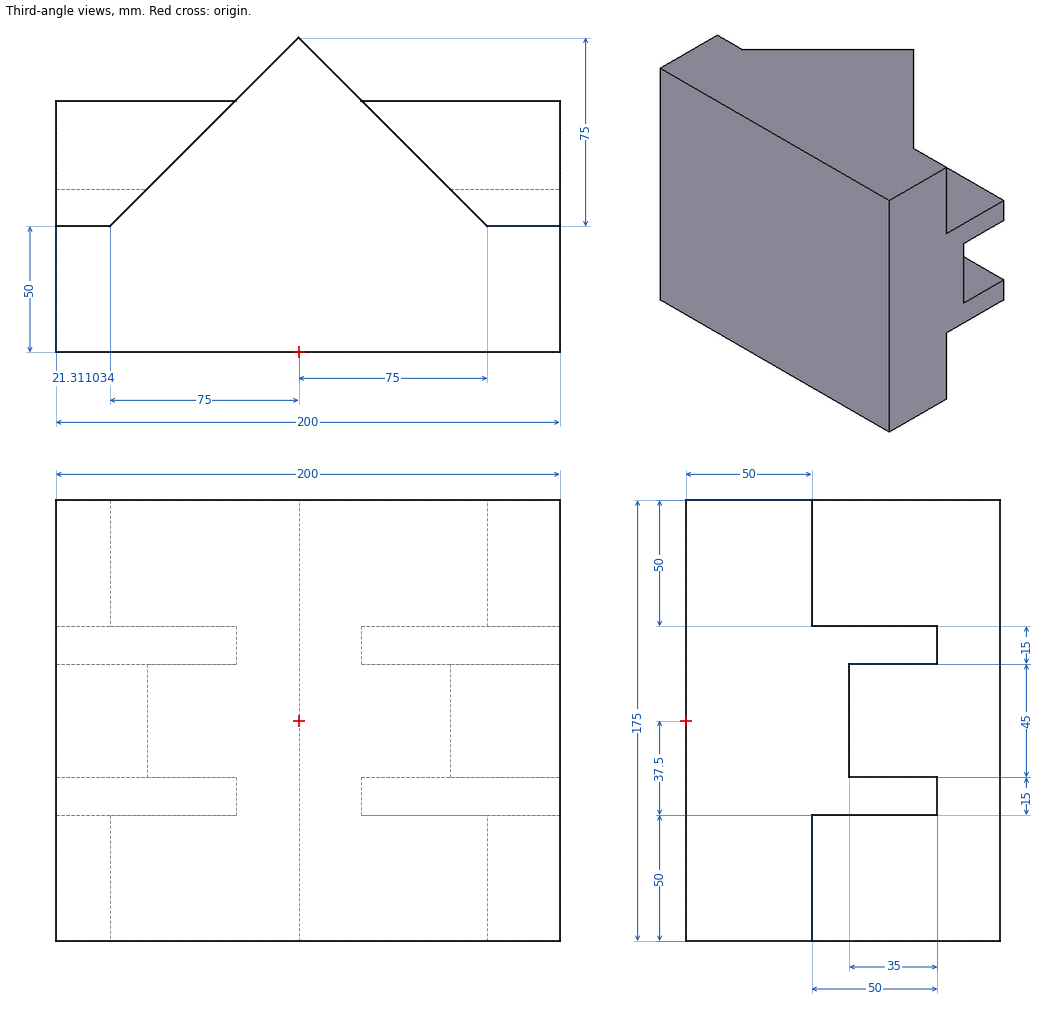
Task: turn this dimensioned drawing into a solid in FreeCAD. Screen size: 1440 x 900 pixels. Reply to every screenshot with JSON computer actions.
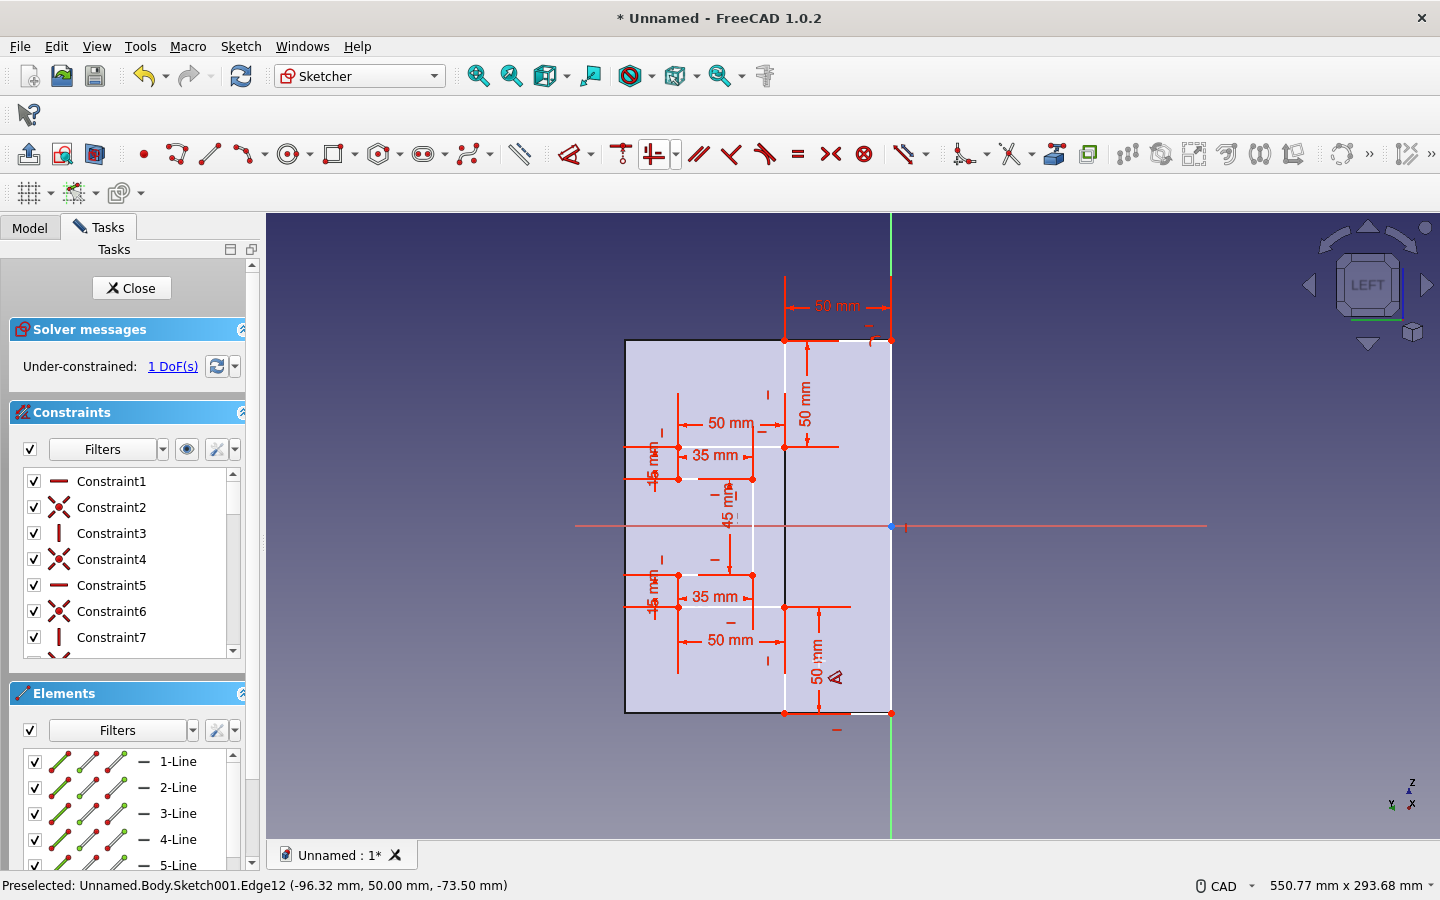
{"action": "left_click", "coordinate": [785, 607]}
{"action": "left_click", "coordinate": [925, 567]}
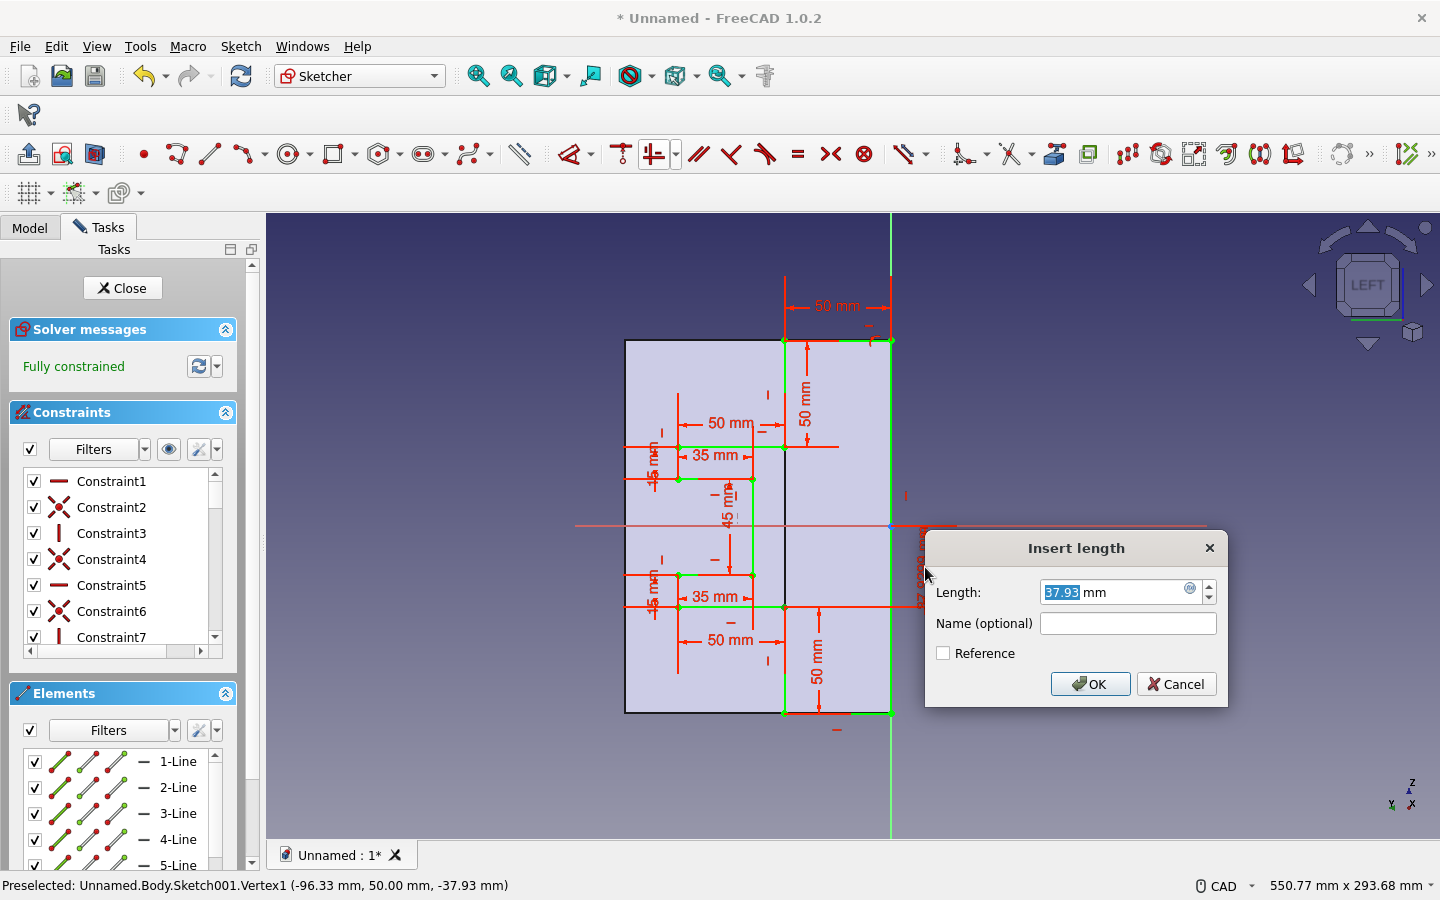
{"action": "type", "text": "37.5"}
{"action": "key", "text": "Return"}
{"action": "key", "text": "Escape"}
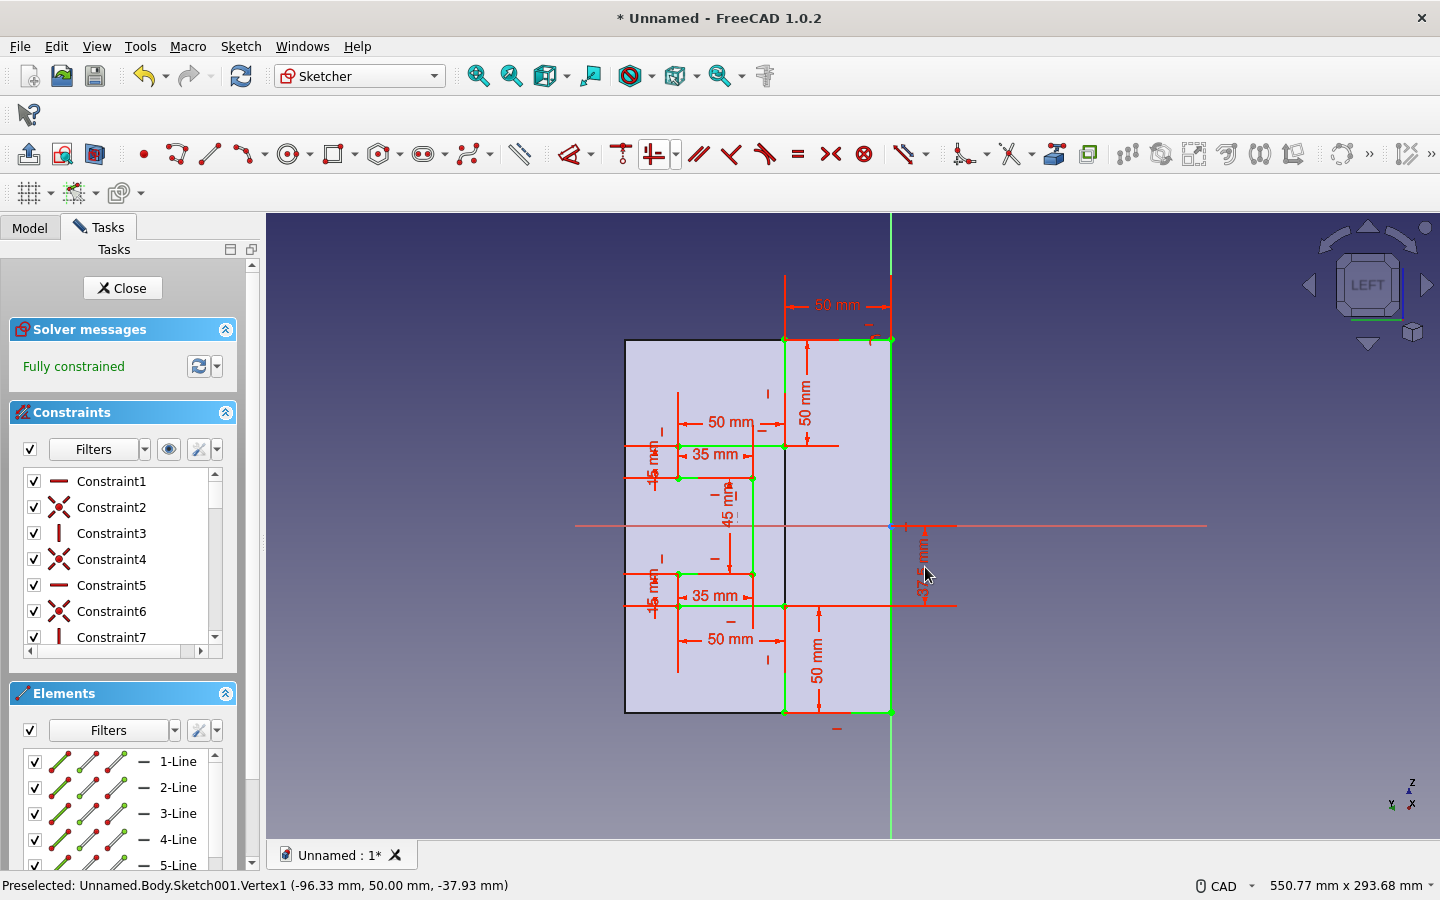
{"action": "left_click", "coordinate": [123, 288]}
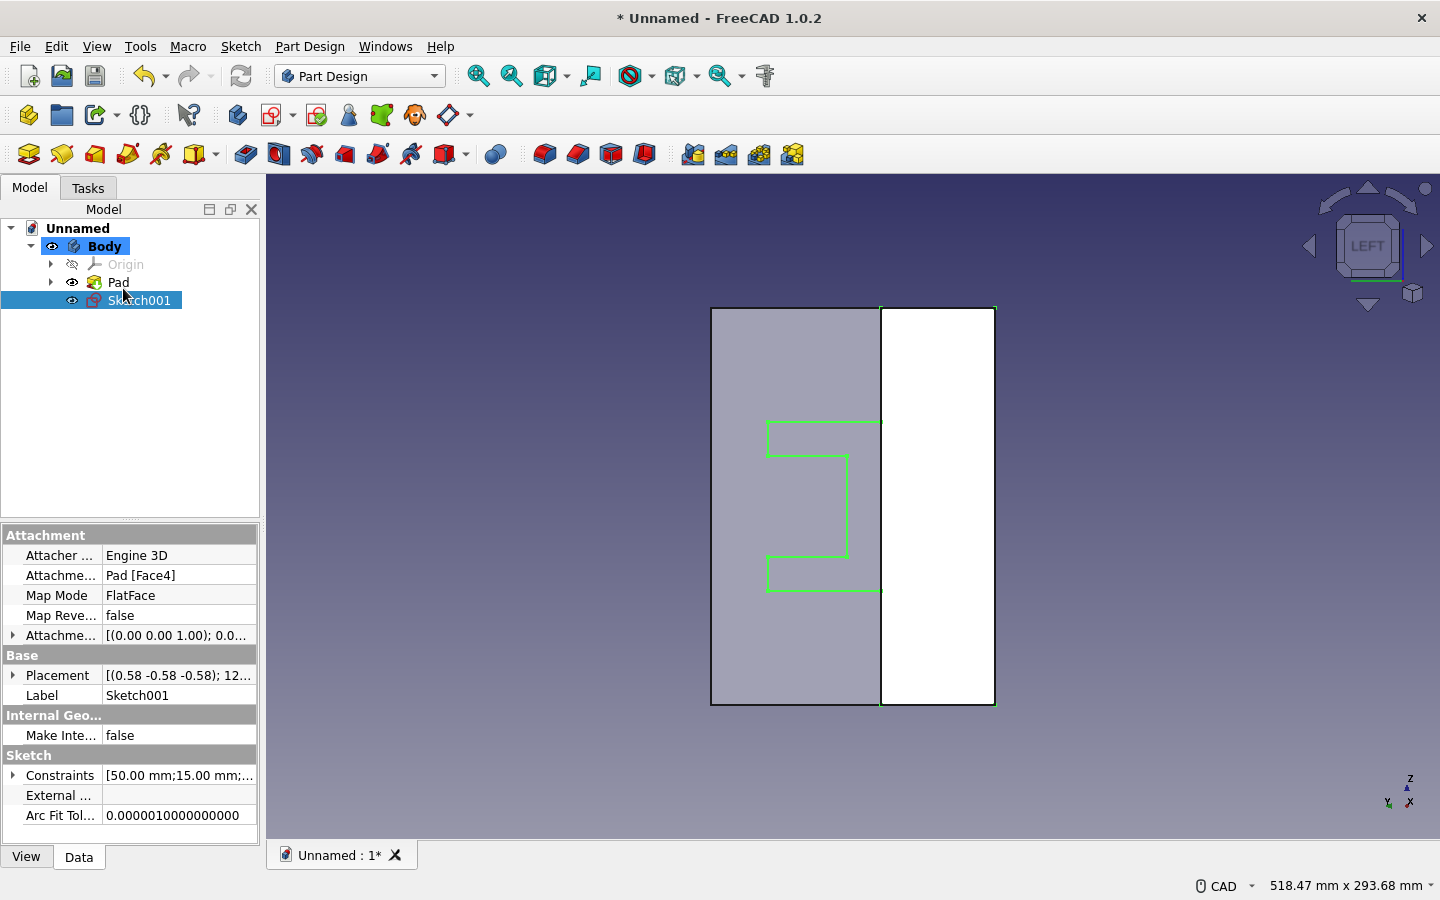
{"action": "left_click", "coordinate": [29, 154]}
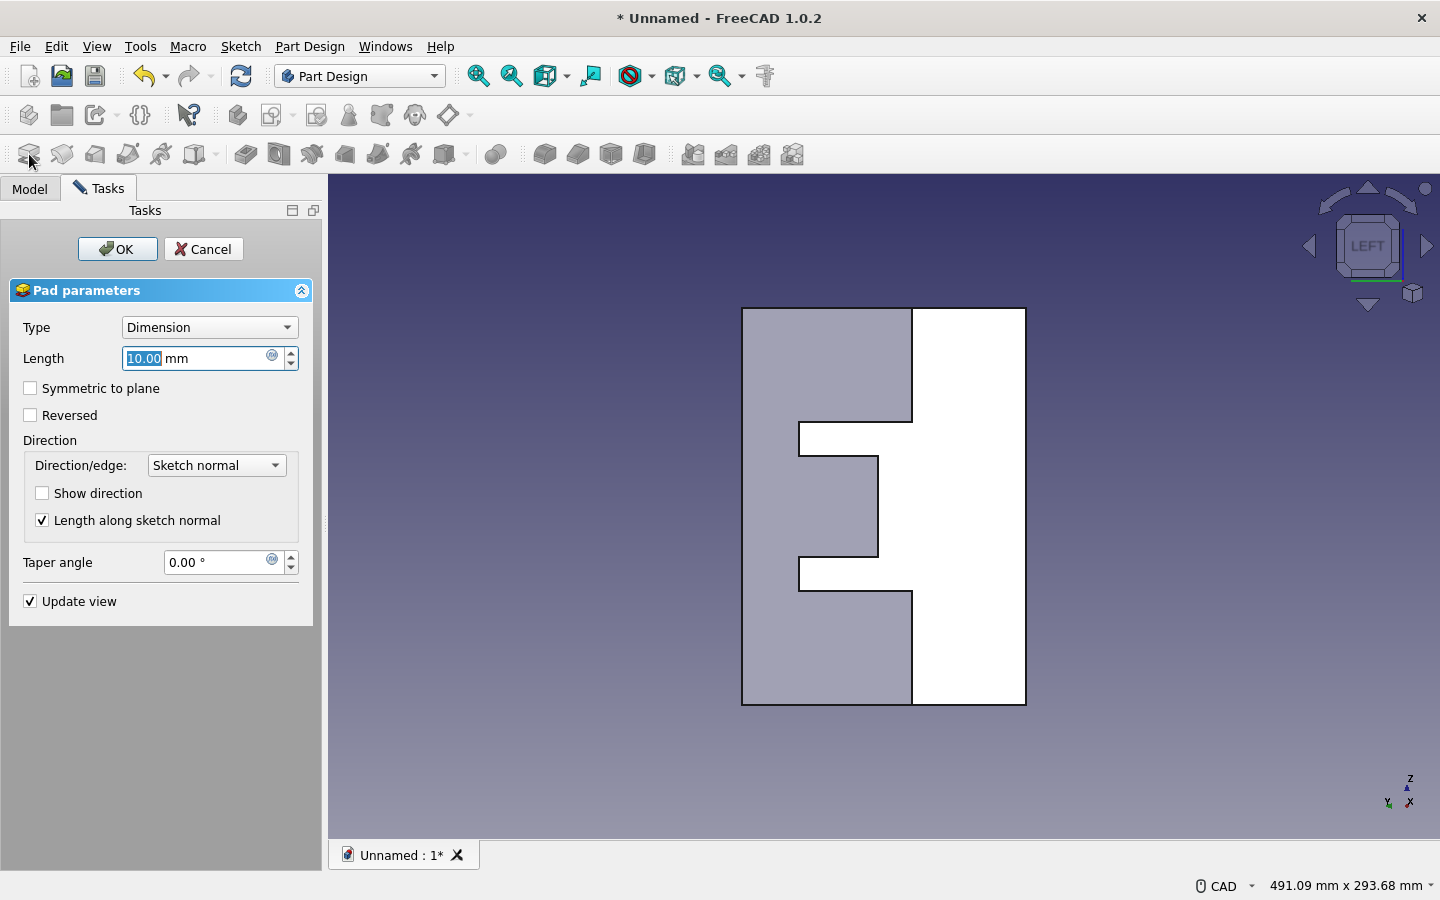
{"action": "type", "text": "200"}
{"action": "key", "text": "Tab"}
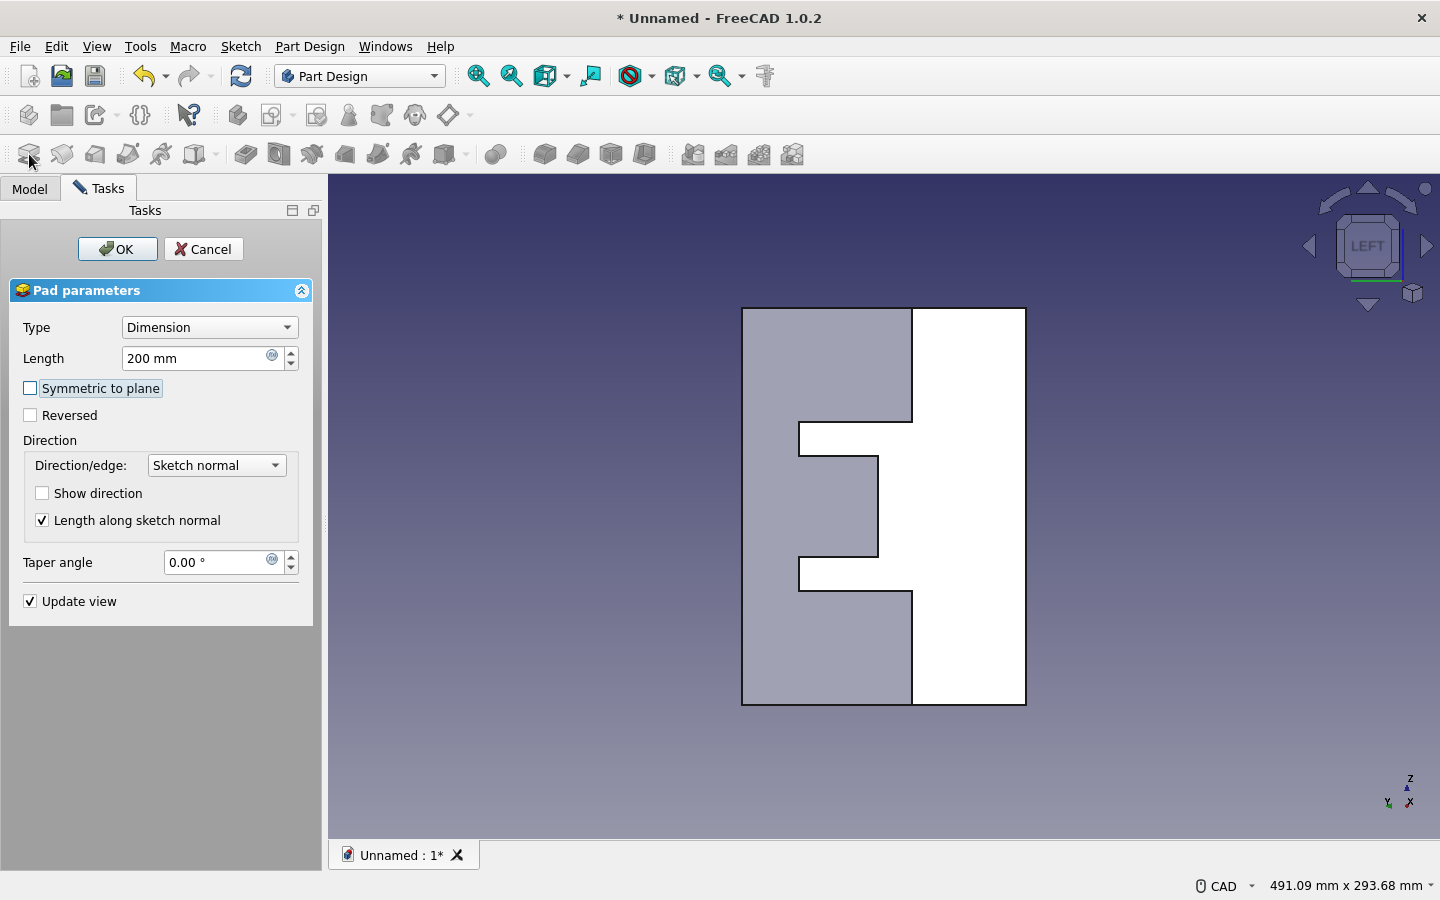
{"action": "left_click", "coordinate": [31, 415]}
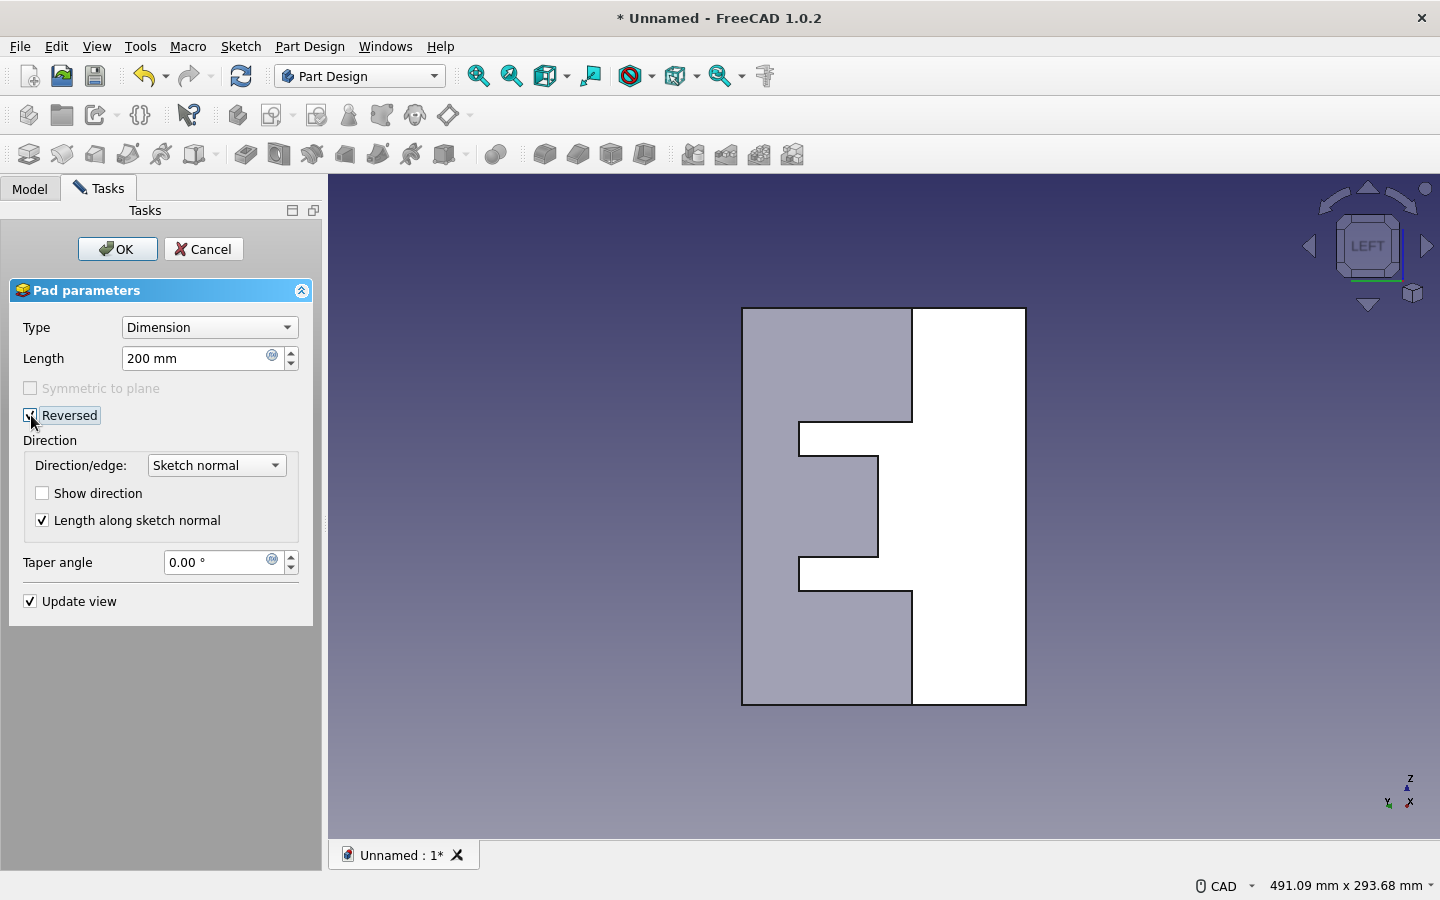
{"action": "left_click", "coordinate": [118, 249]}